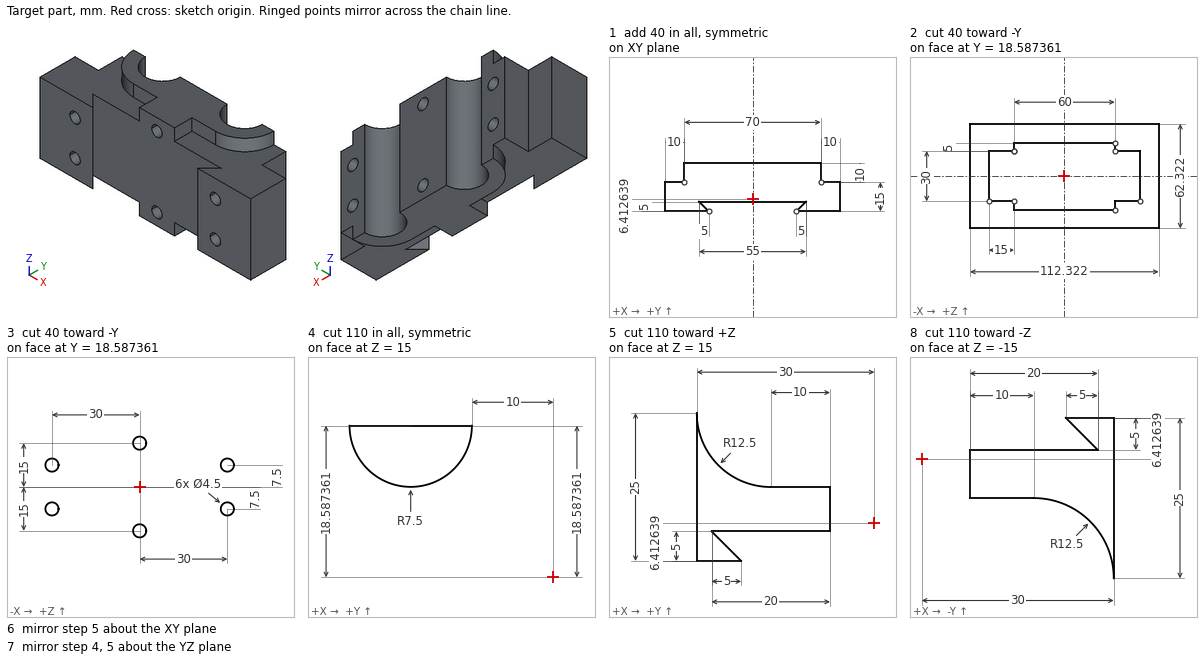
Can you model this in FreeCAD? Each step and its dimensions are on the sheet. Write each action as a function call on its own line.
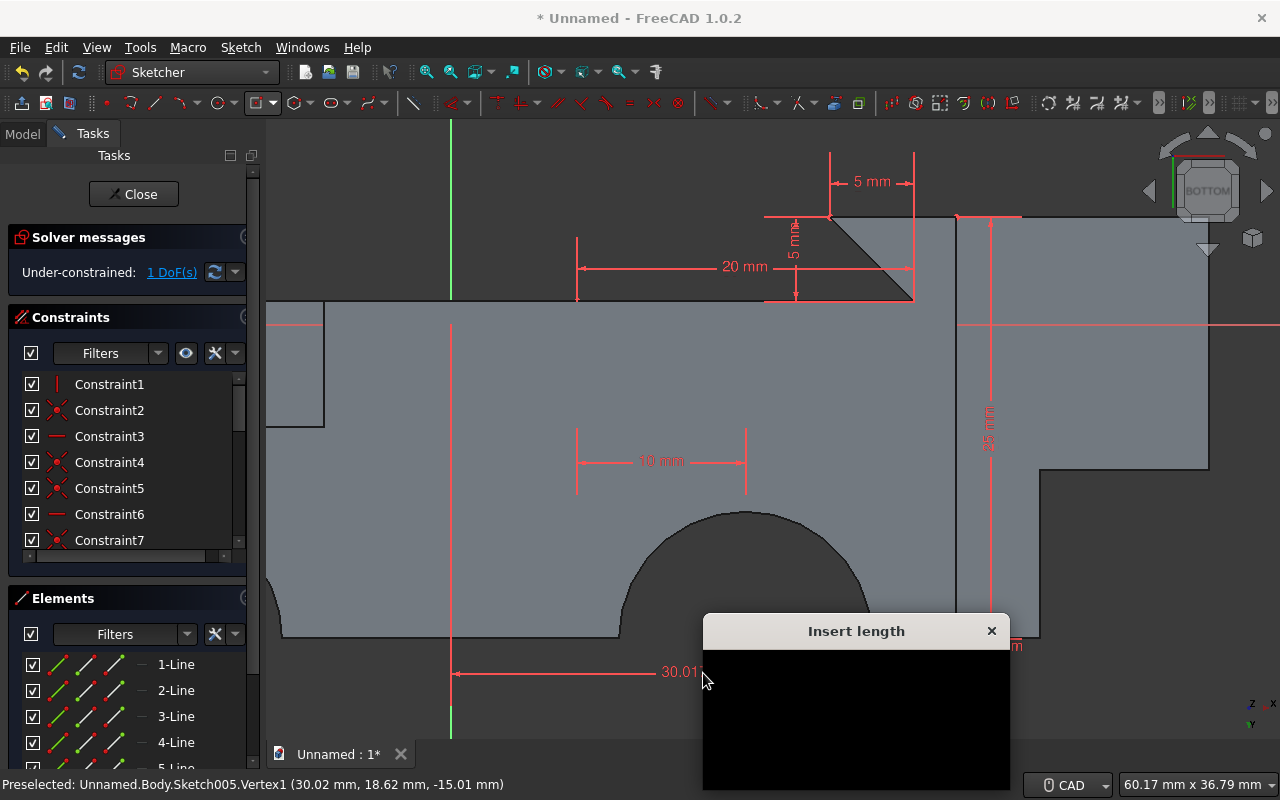
text(30)
key(Return)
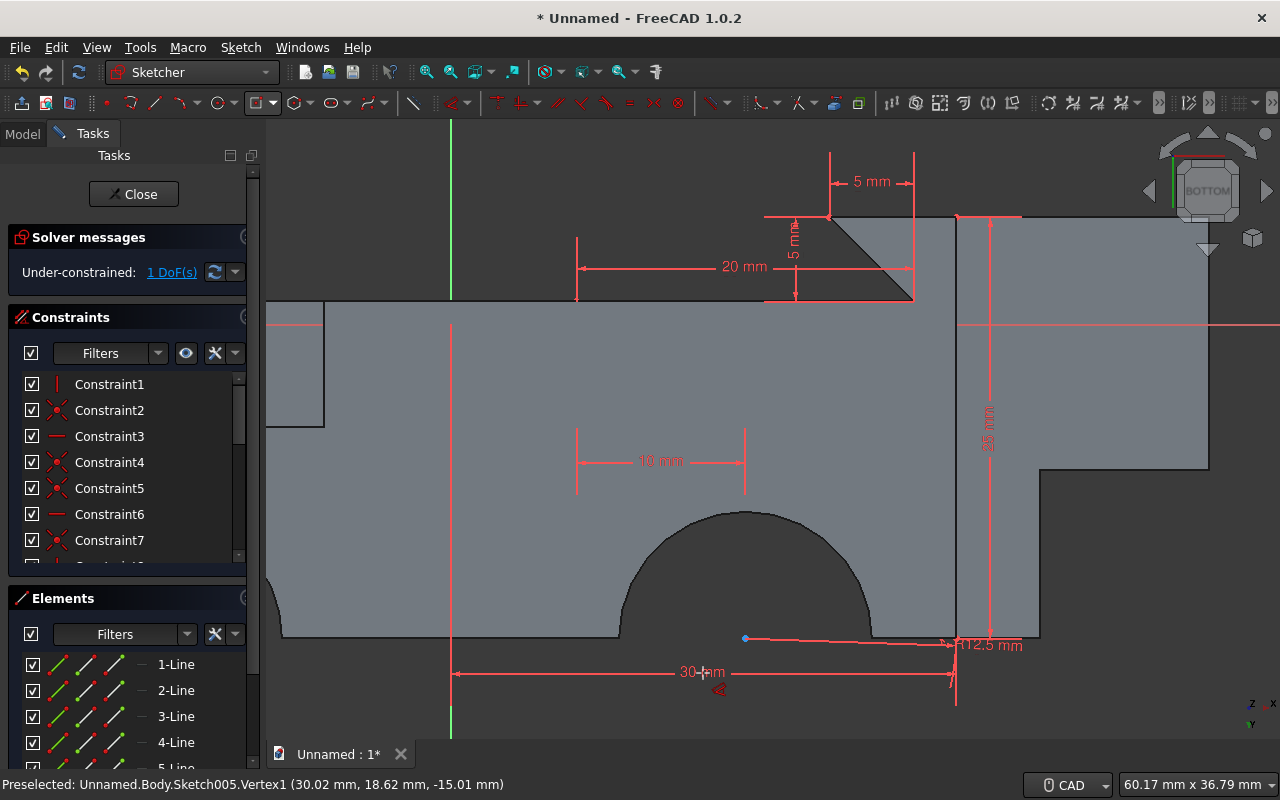
click(956, 217)
click(990, 271)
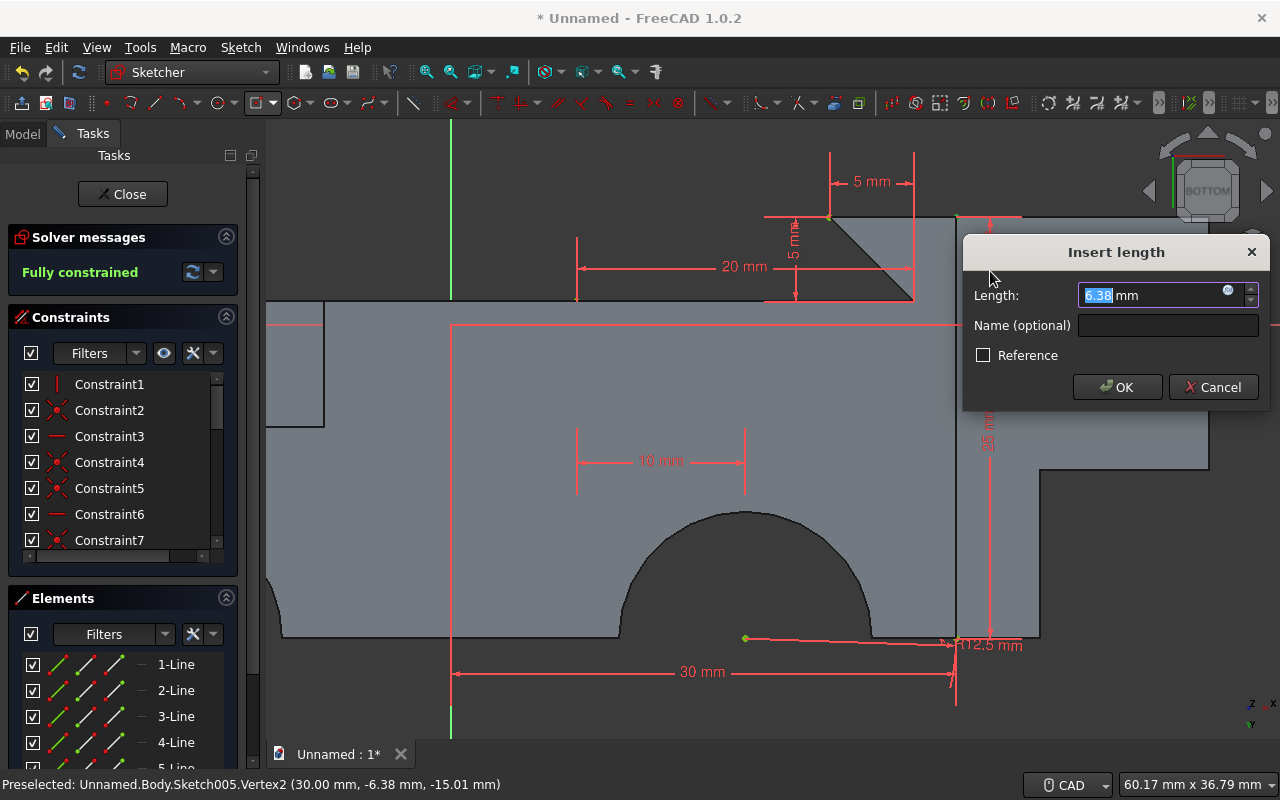
text(6.412639)
key(Return)
key(Escape)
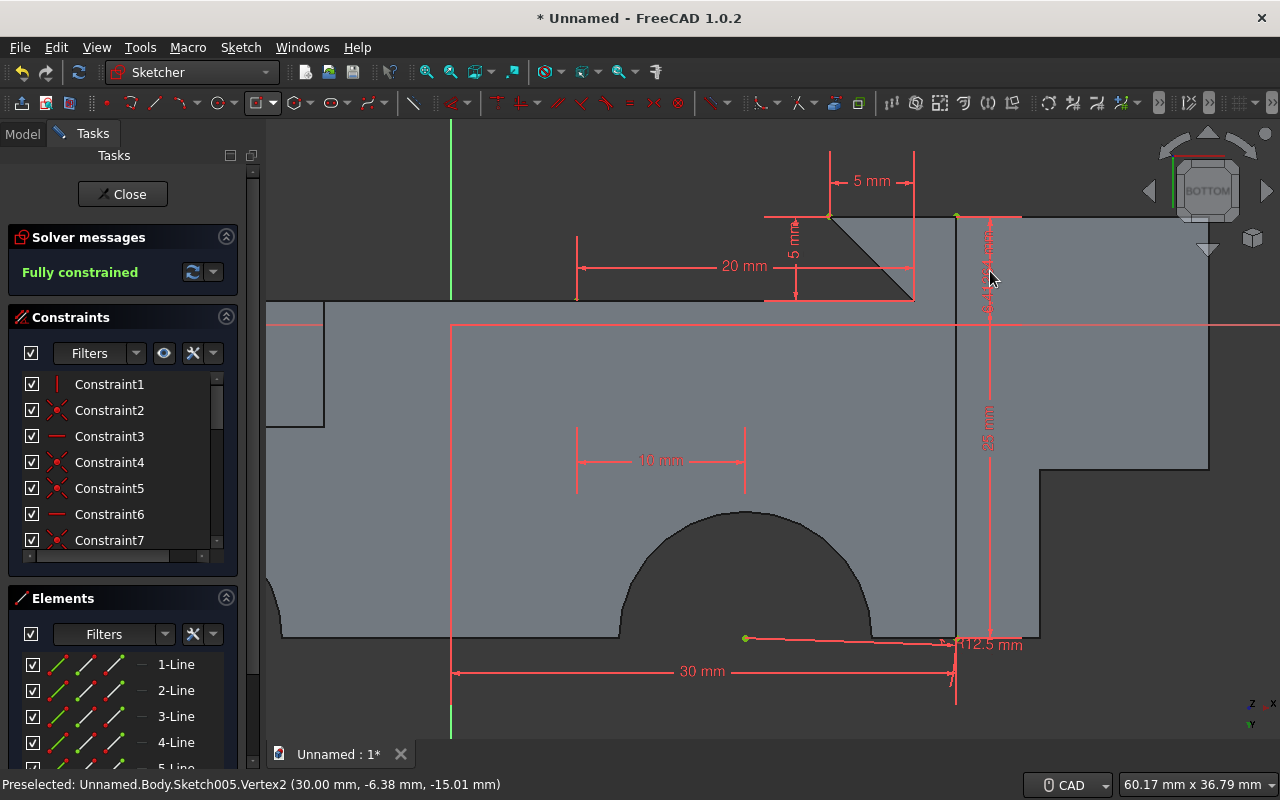
click(123, 194)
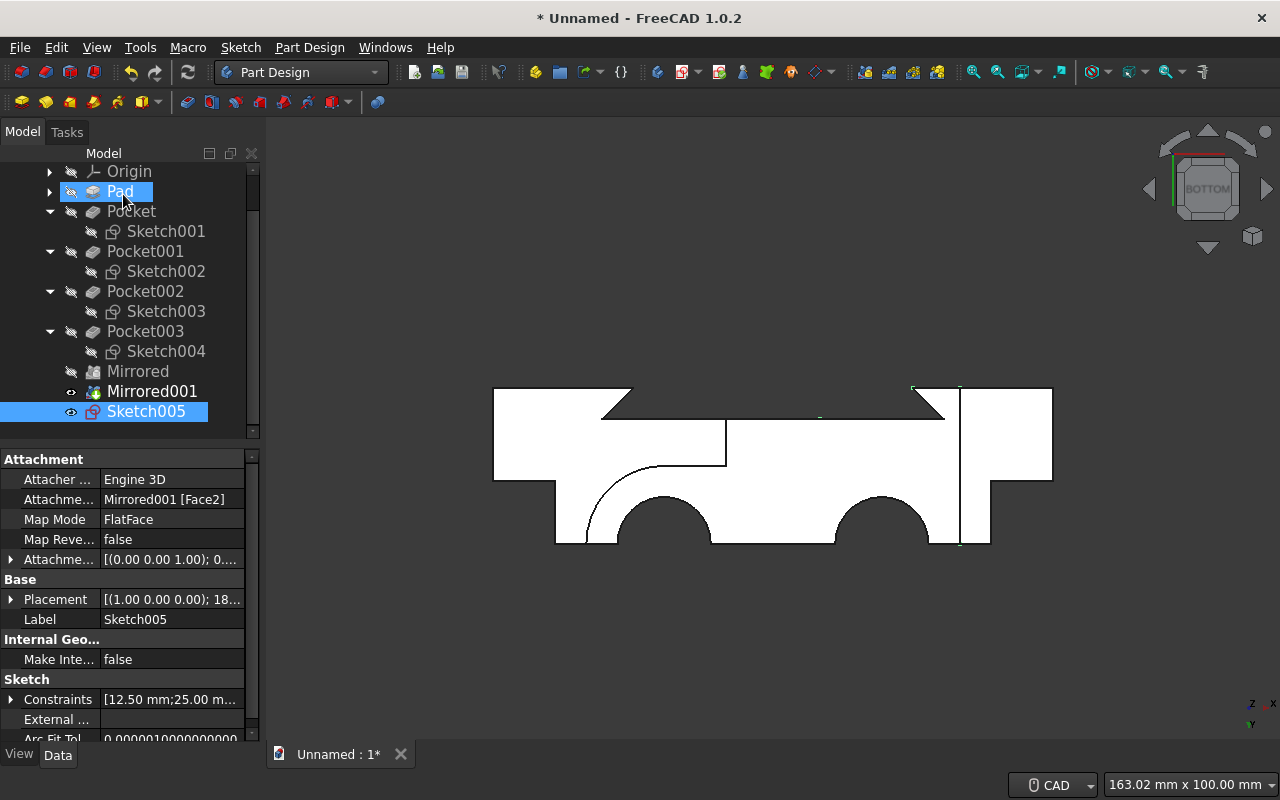
click(188, 102)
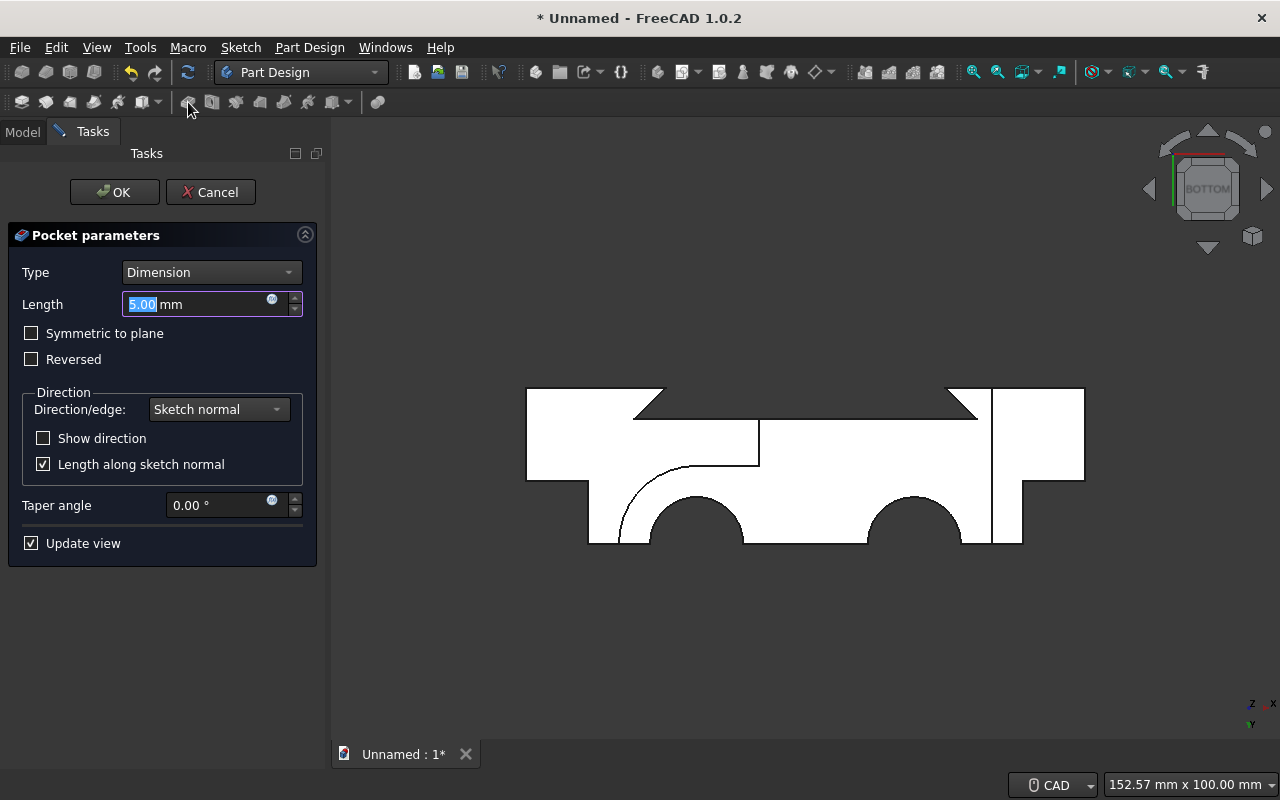
text(110)
key(Tab)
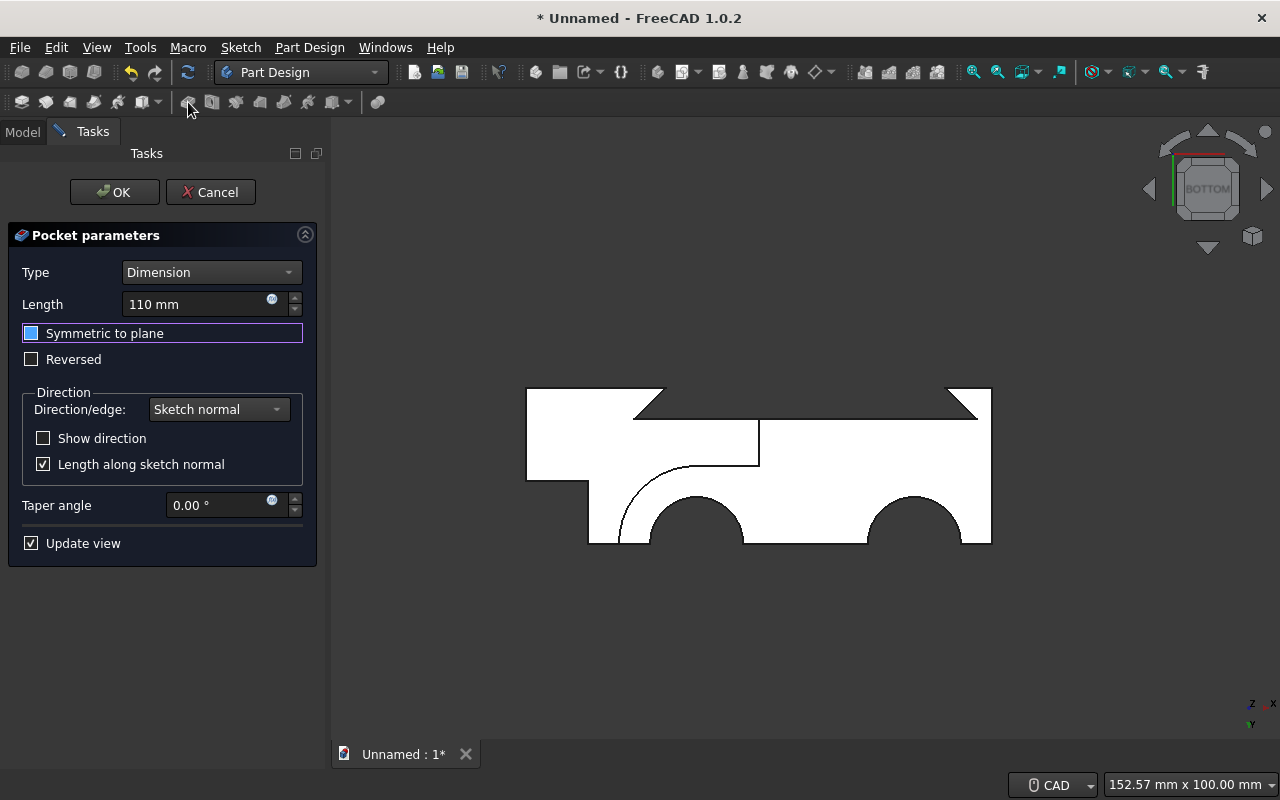
click(30, 359)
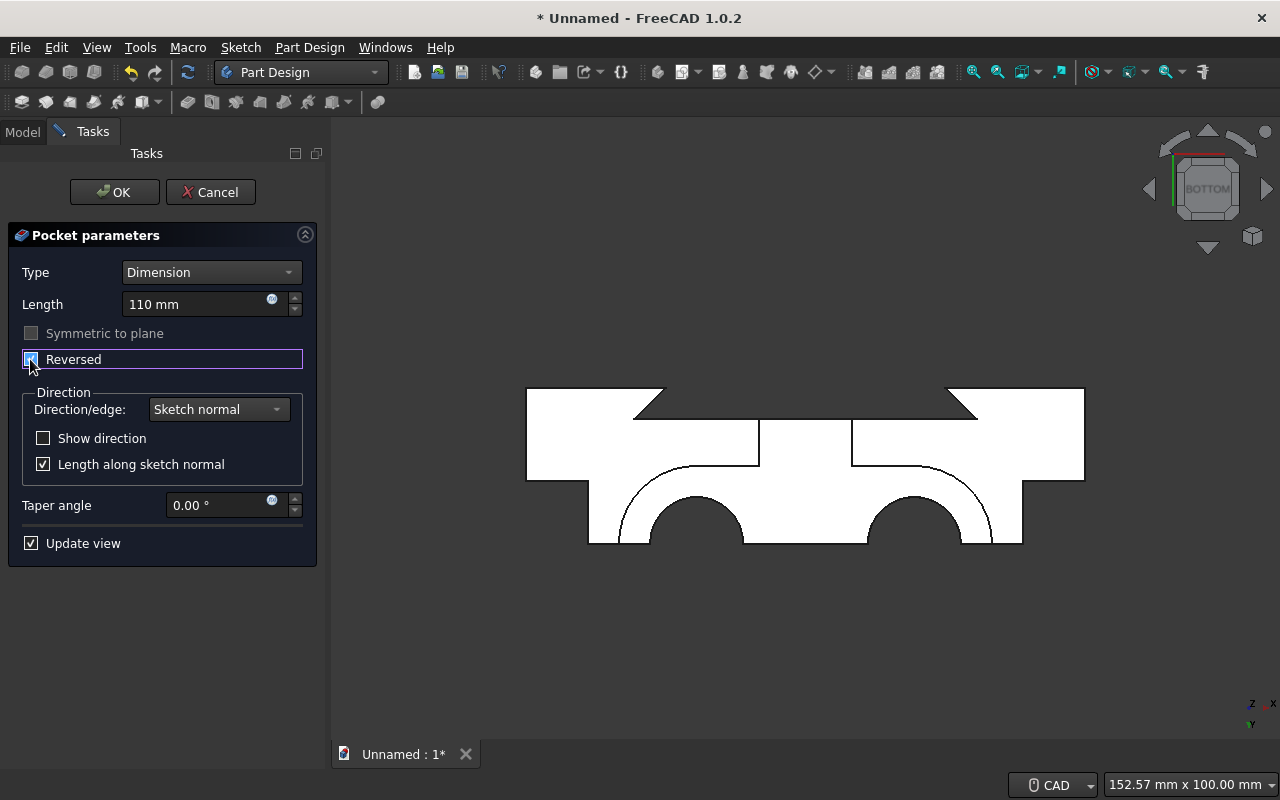
click(115, 192)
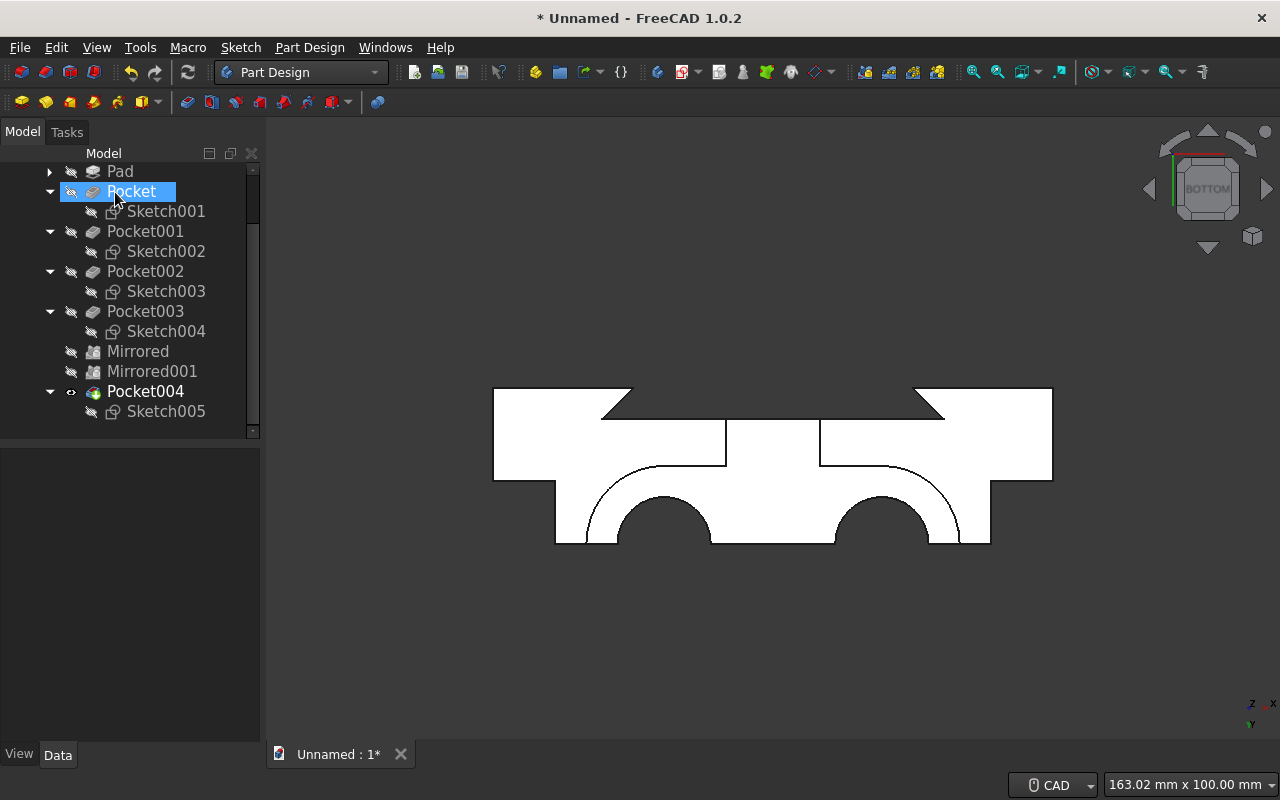
key(0)